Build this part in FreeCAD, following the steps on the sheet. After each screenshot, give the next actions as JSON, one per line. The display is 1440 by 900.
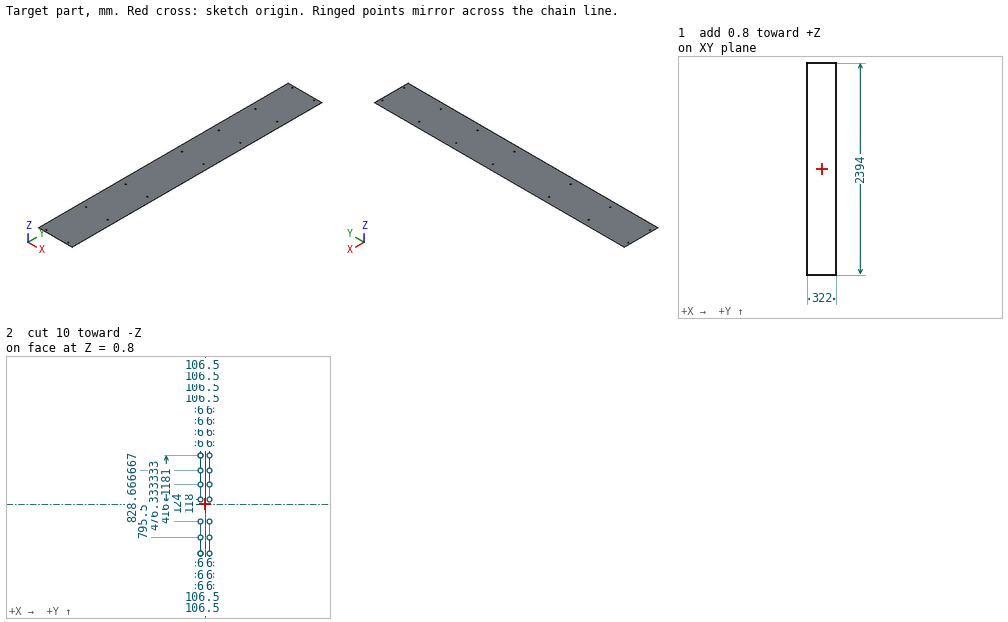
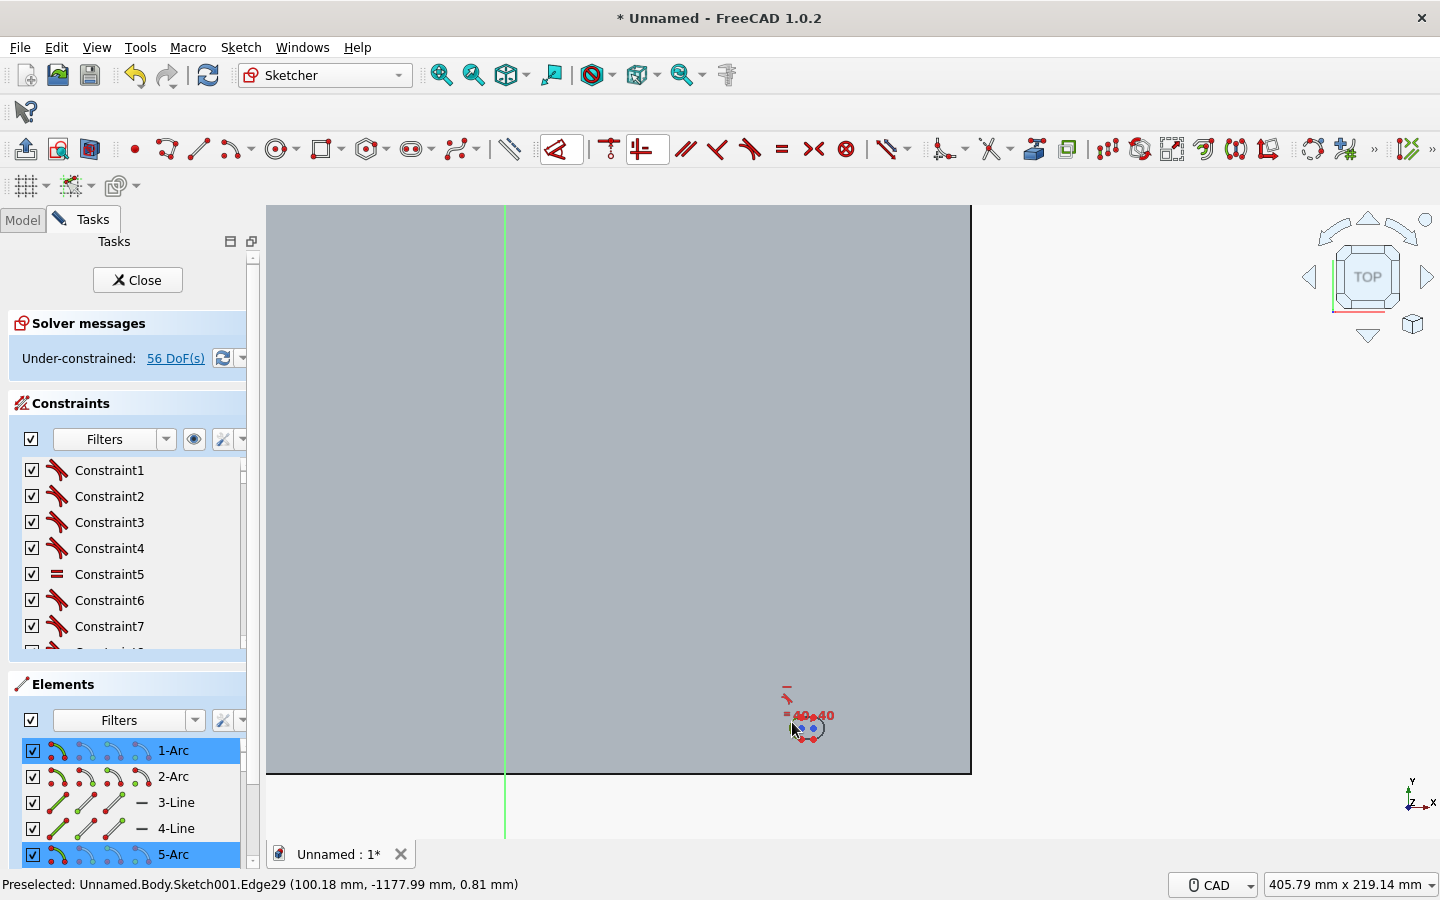
{"action": "scroll", "coordinate": [803, 730], "scroll_direction": "down", "scroll_amount": 14}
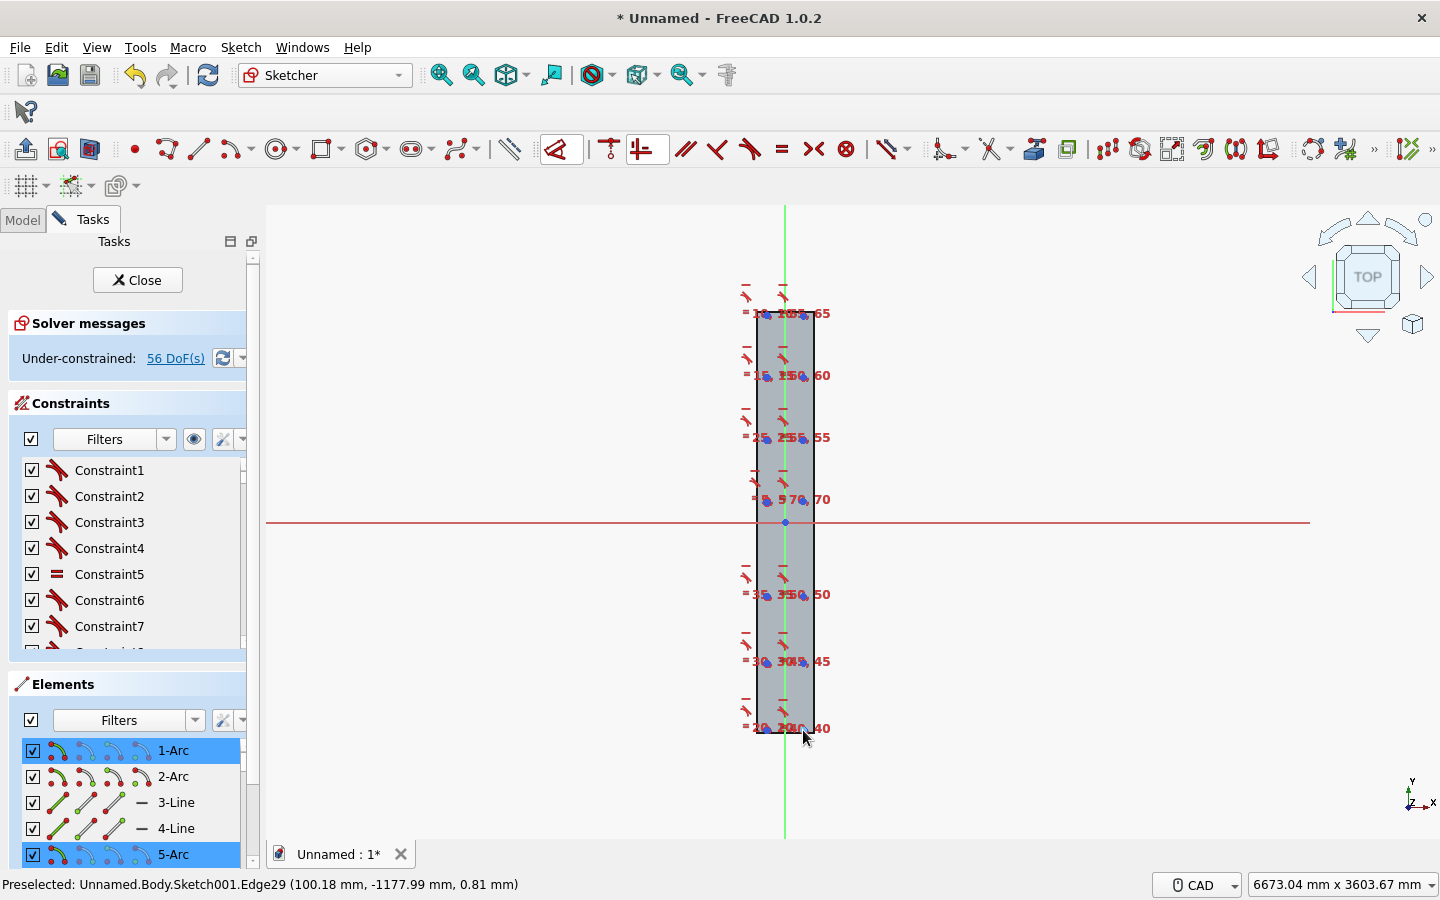
{"action": "scroll", "coordinate": [803, 663], "scroll_direction": "up", "scroll_amount": 14}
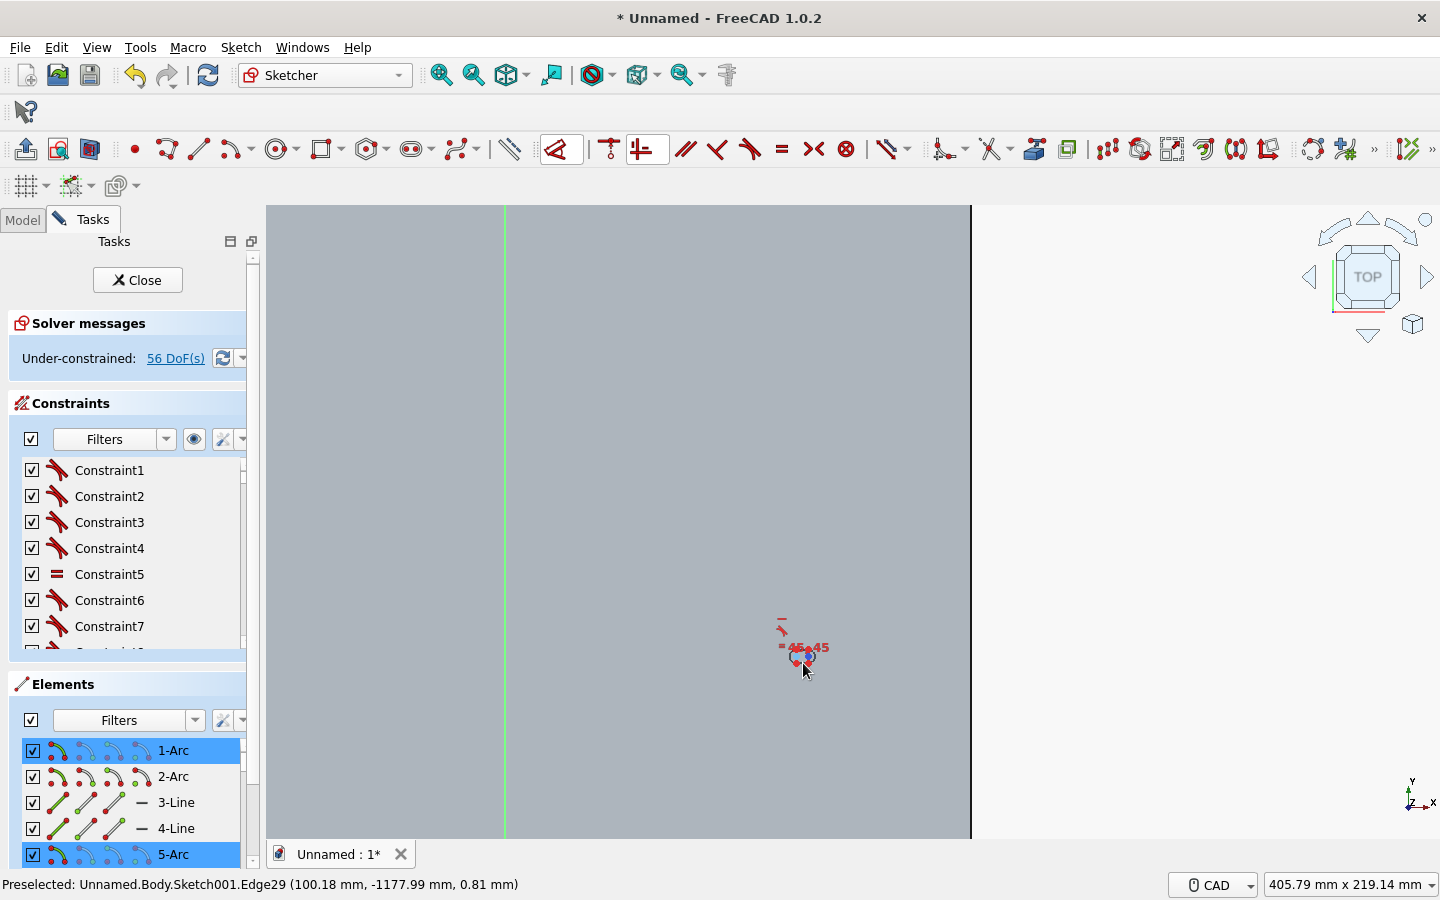
{"action": "left_click", "coordinate": [790, 656]}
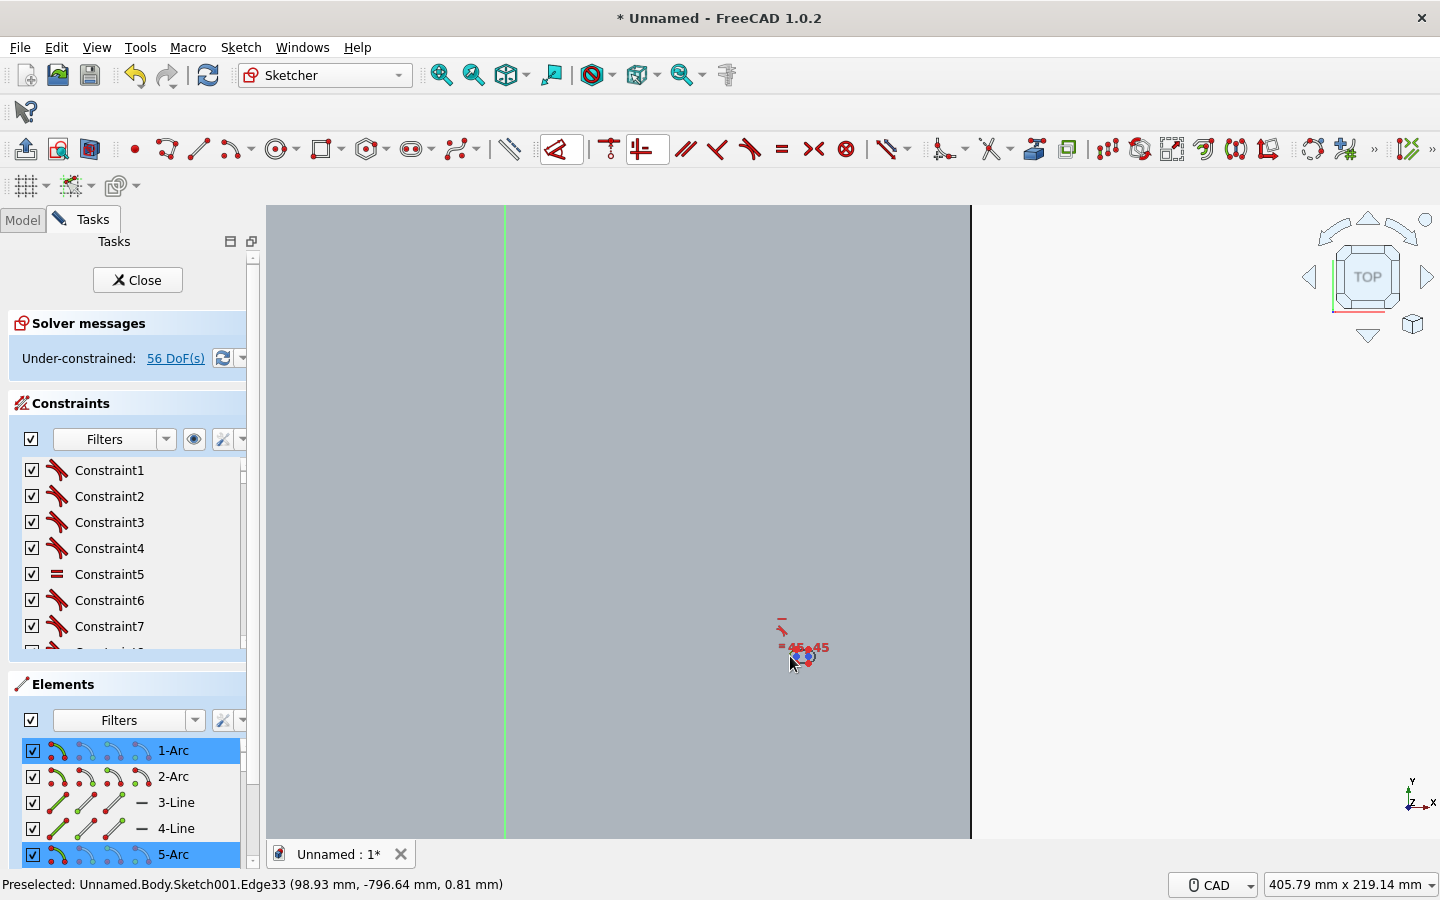
{"action": "scroll", "coordinate": [803, 663], "scroll_direction": "down", "scroll_amount": 14}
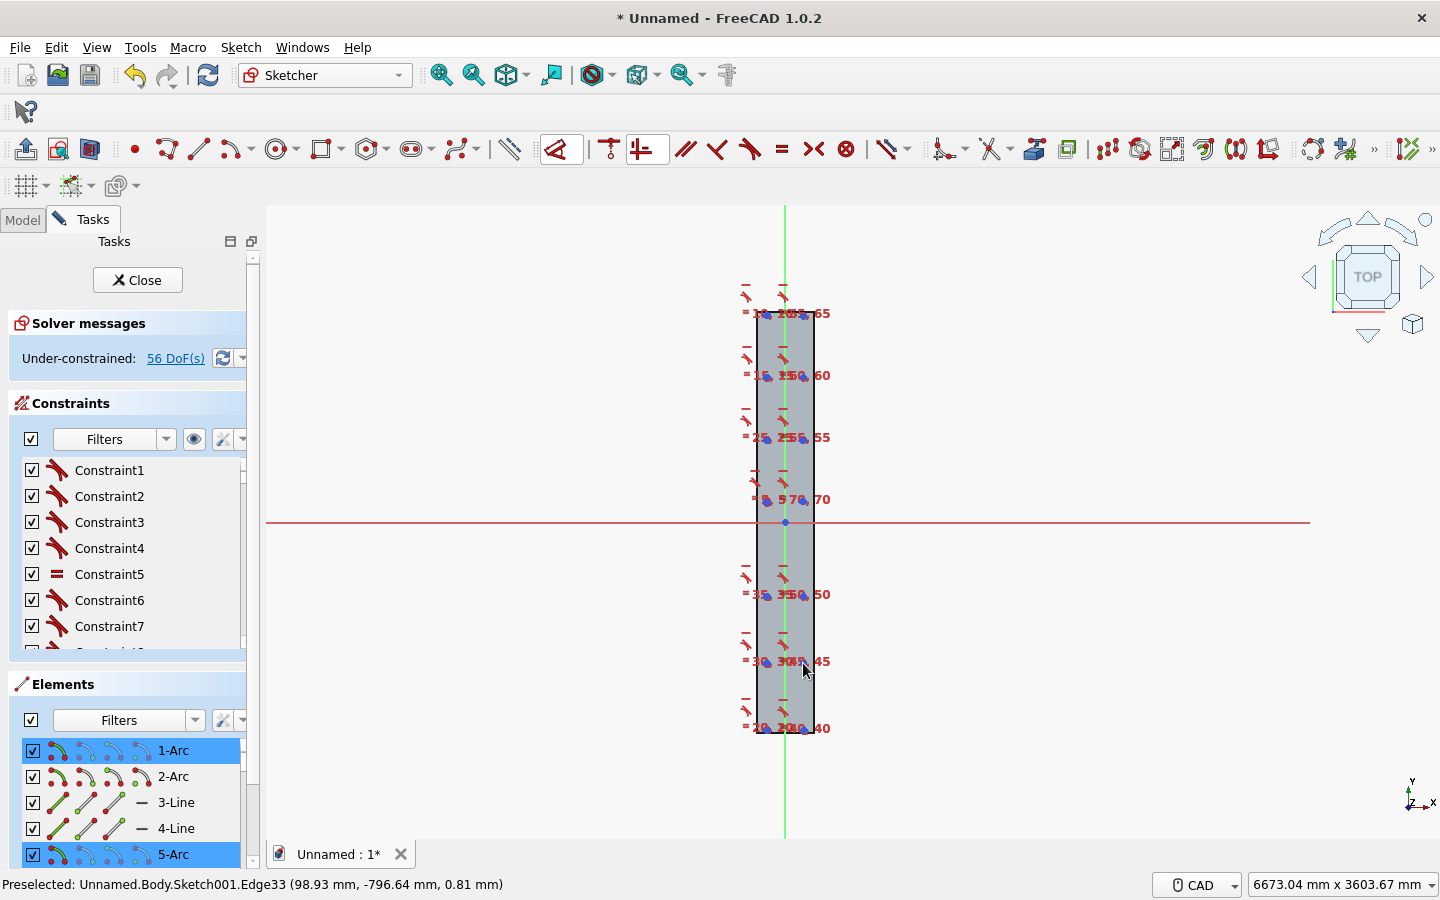
{"action": "scroll", "coordinate": [803, 597], "scroll_direction": "up", "scroll_amount": 14}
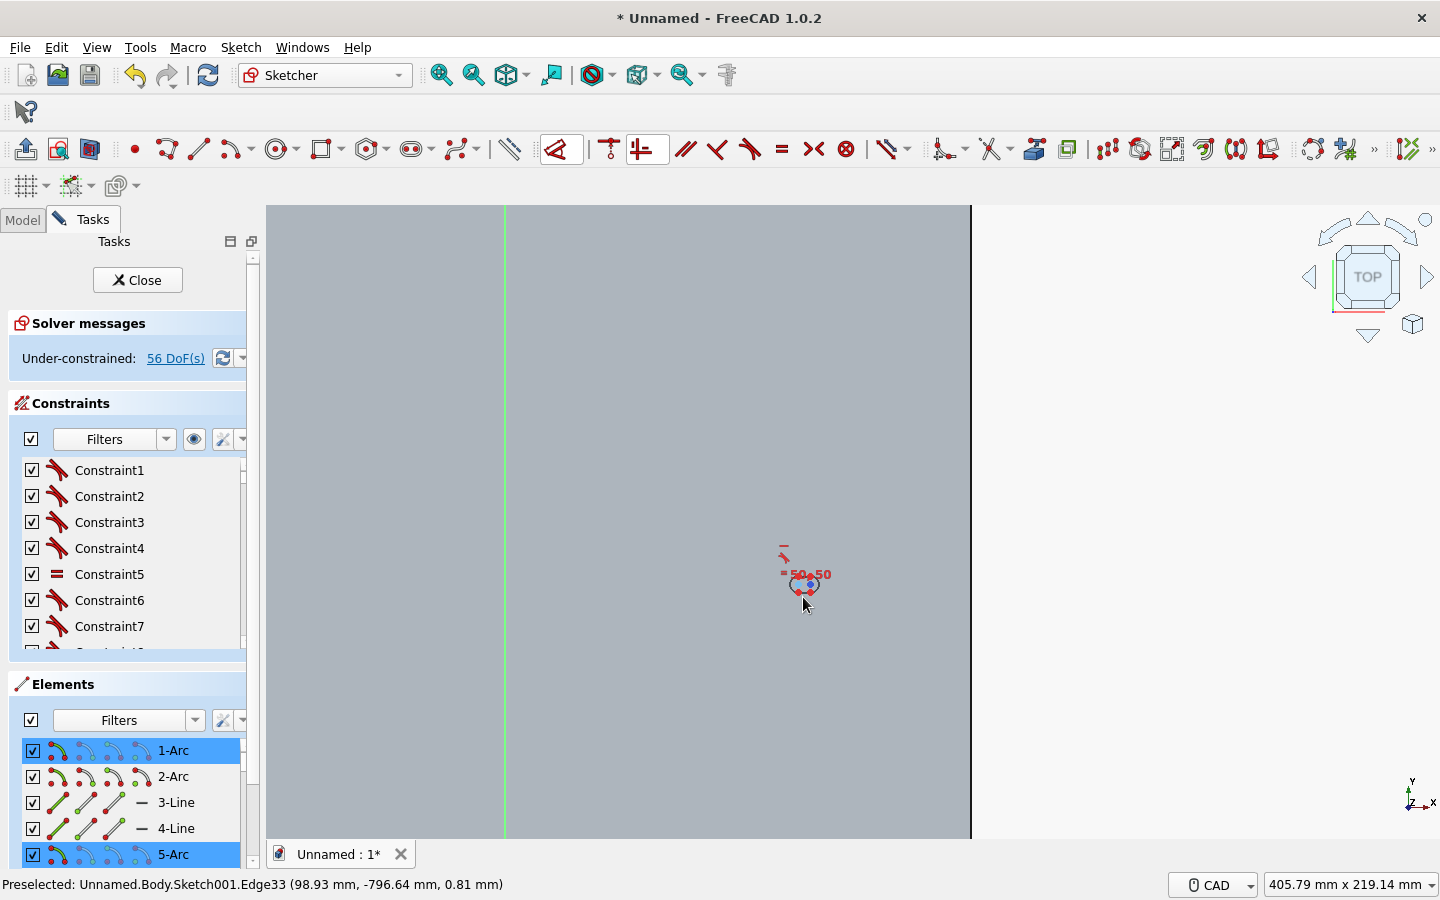
{"action": "left_click", "coordinate": [790, 585]}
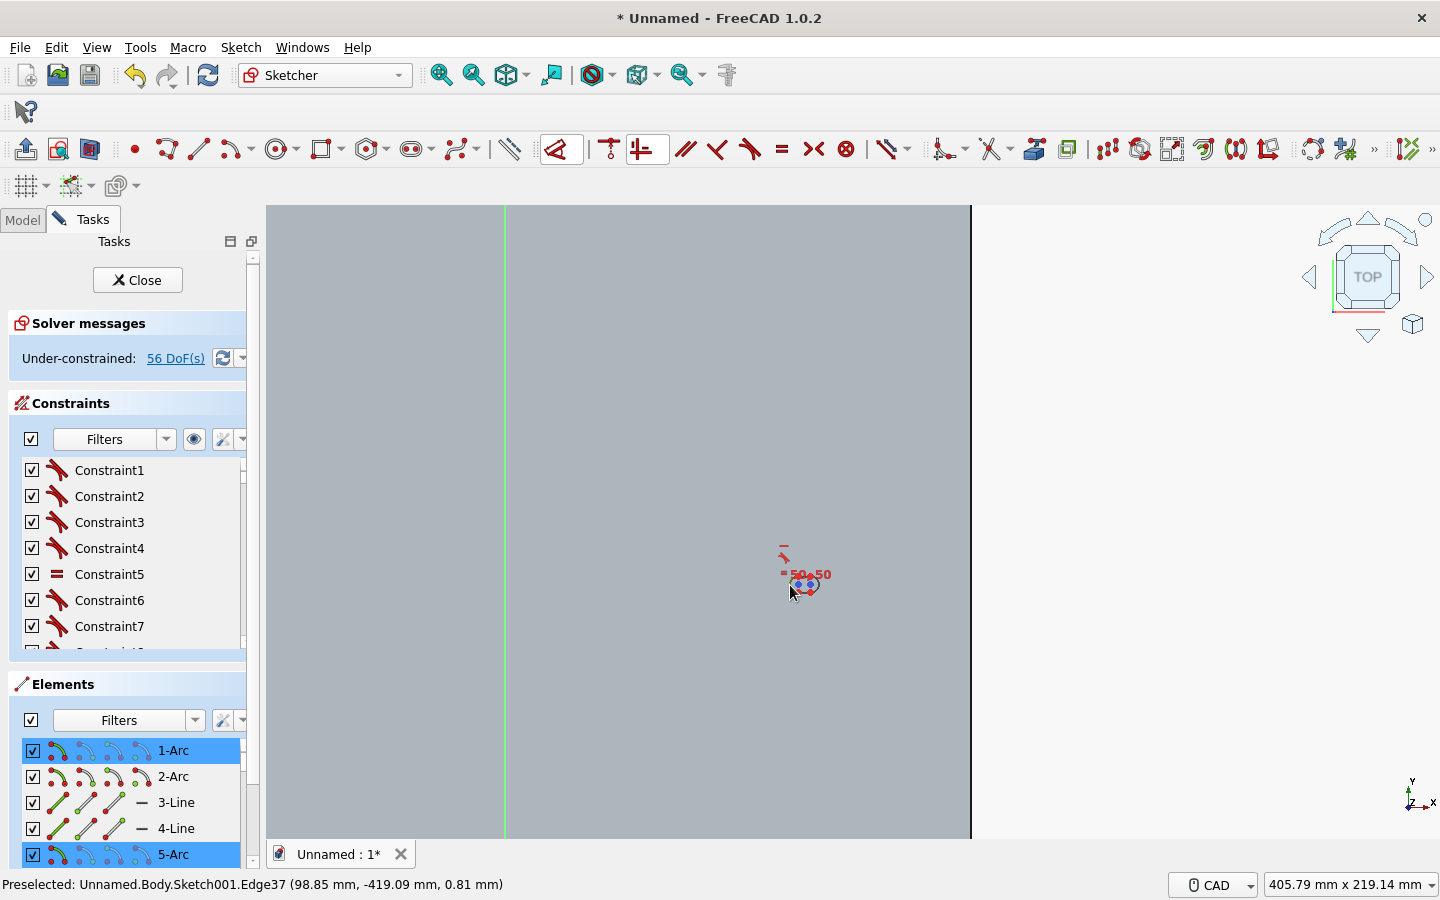
{"action": "scroll", "coordinate": [803, 597], "scroll_direction": "down", "scroll_amount": 14}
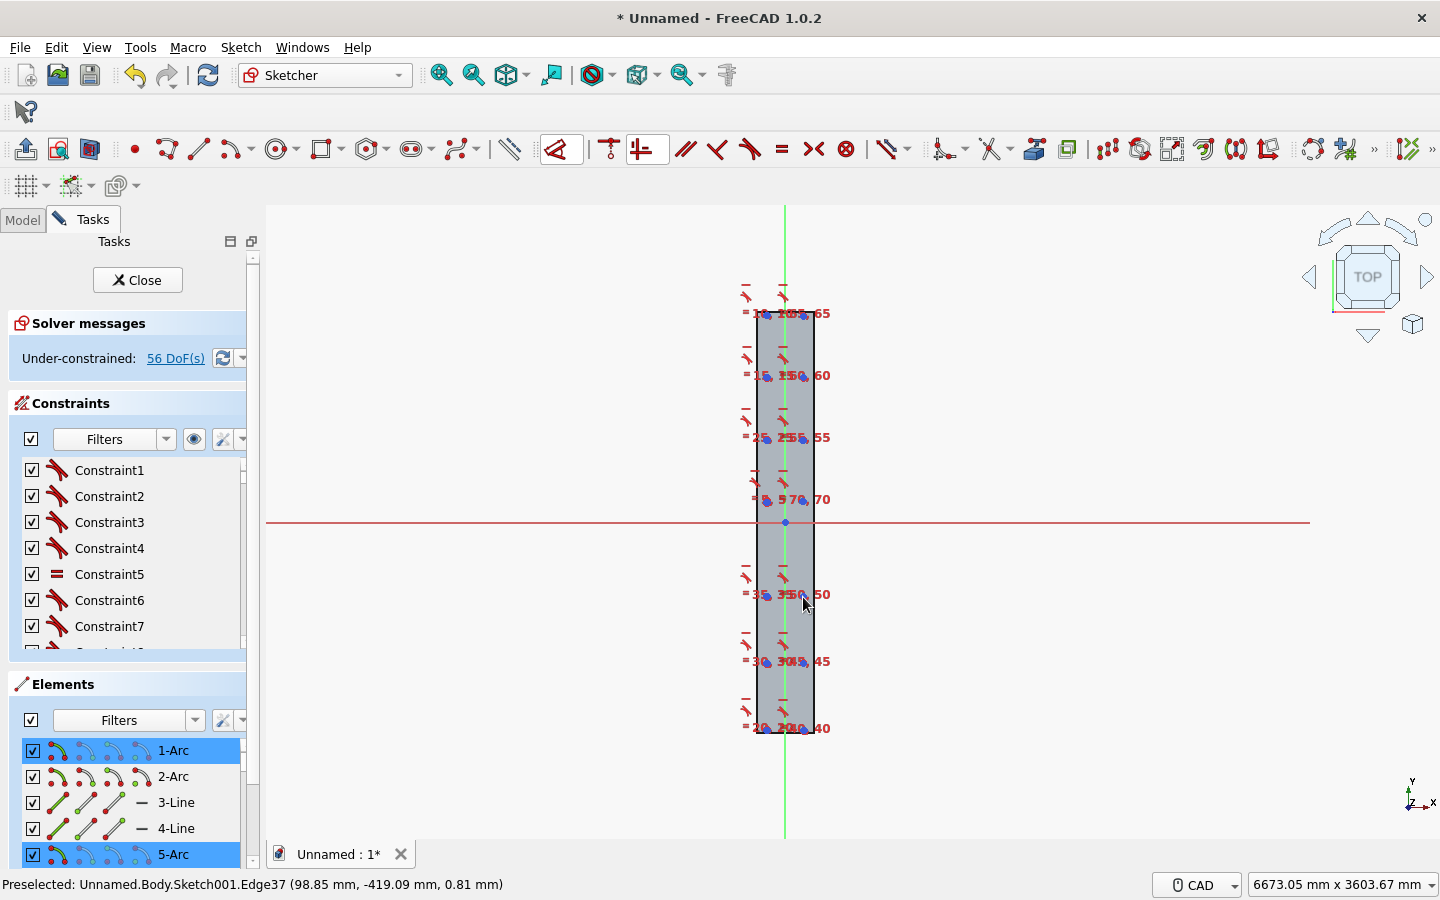
{"action": "scroll", "coordinate": [802, 440], "scroll_direction": "up", "scroll_amount": 14}